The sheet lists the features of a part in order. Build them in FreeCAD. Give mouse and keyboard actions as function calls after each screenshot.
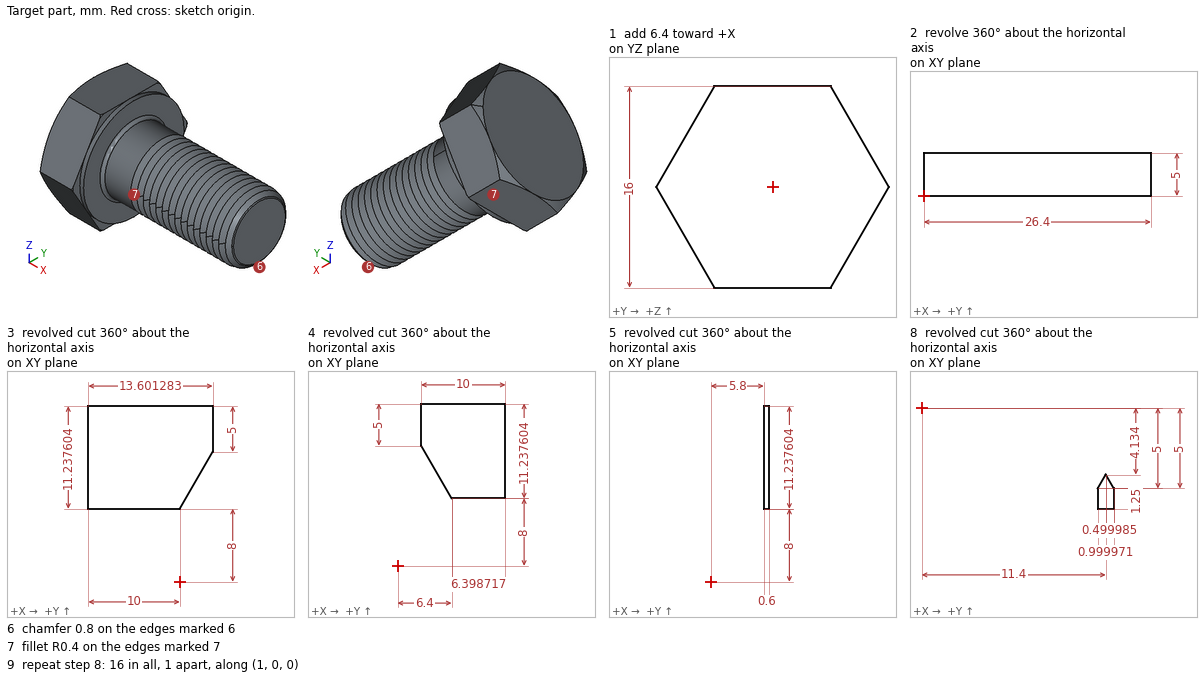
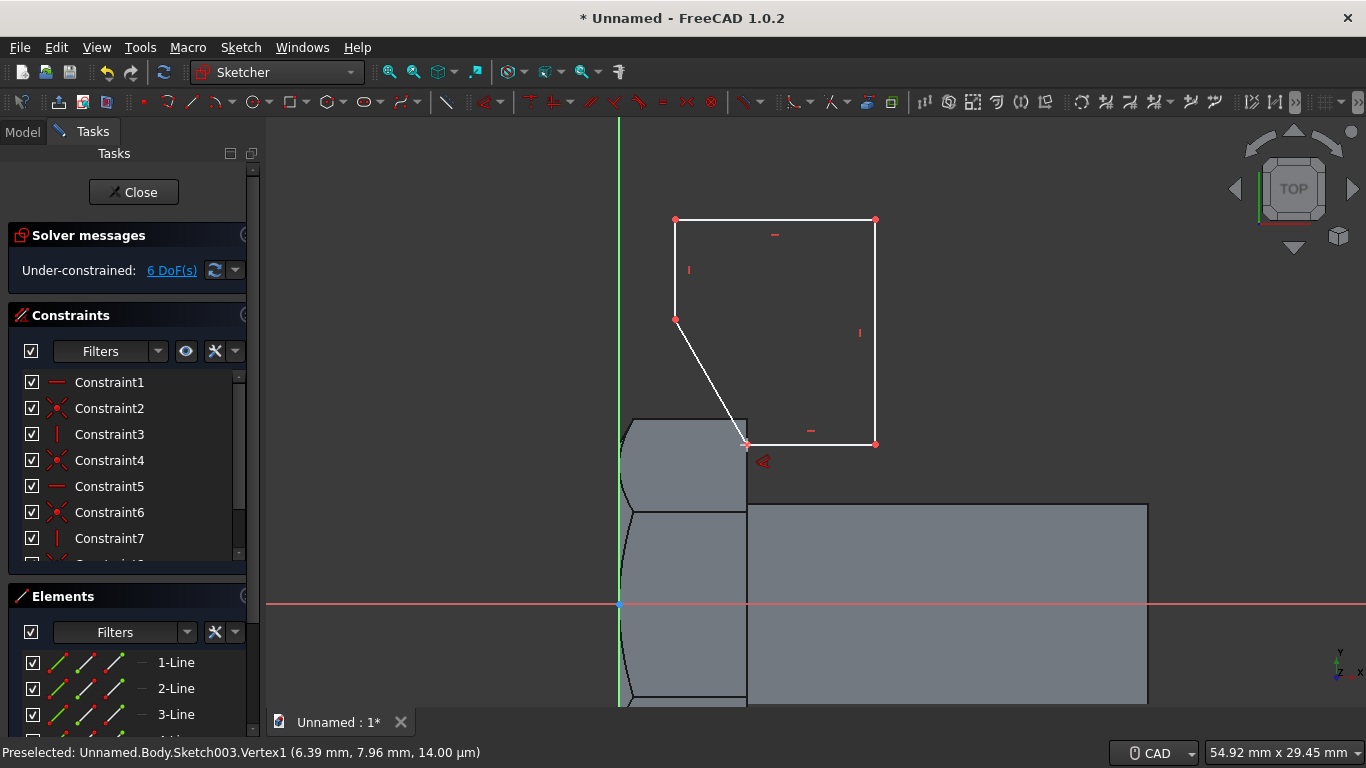
click(675, 250)
click(641, 270)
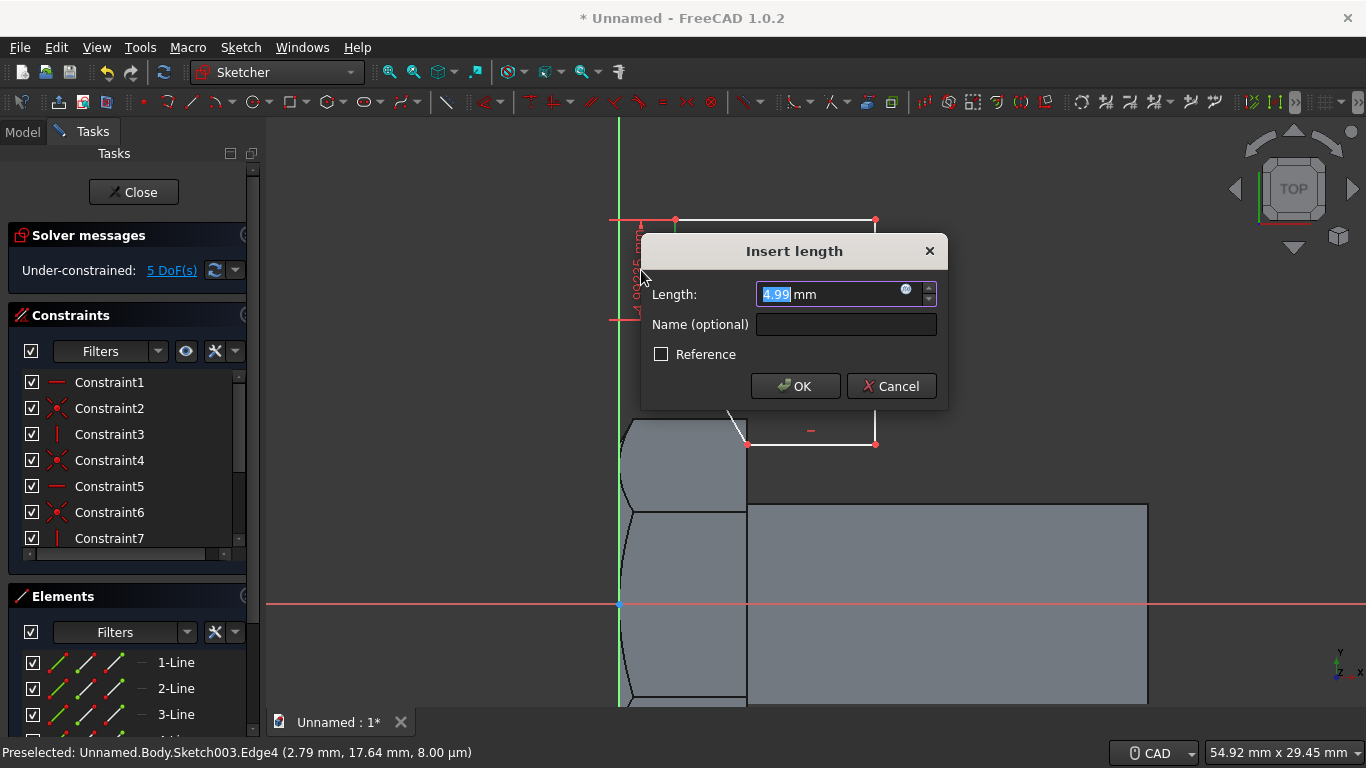
text(5)
key(Return)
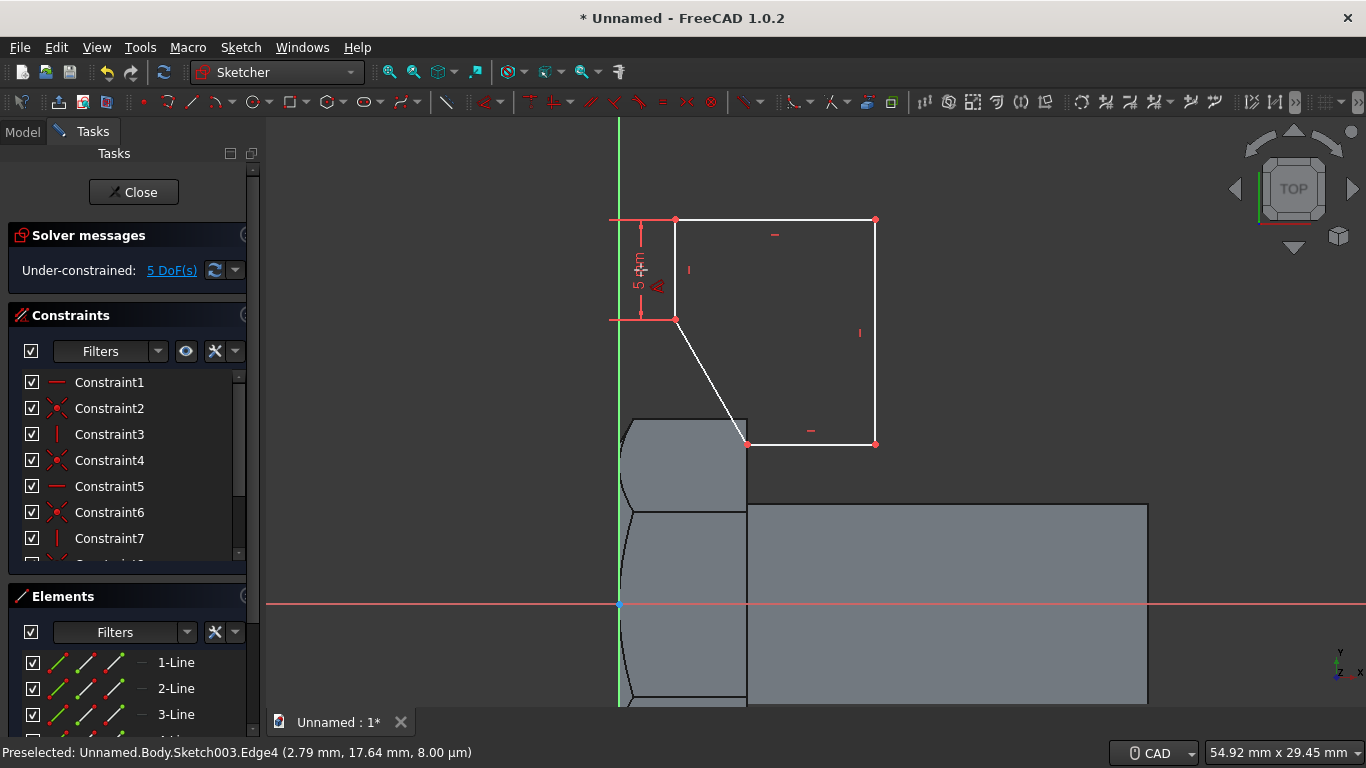
click(815, 220)
click(775, 186)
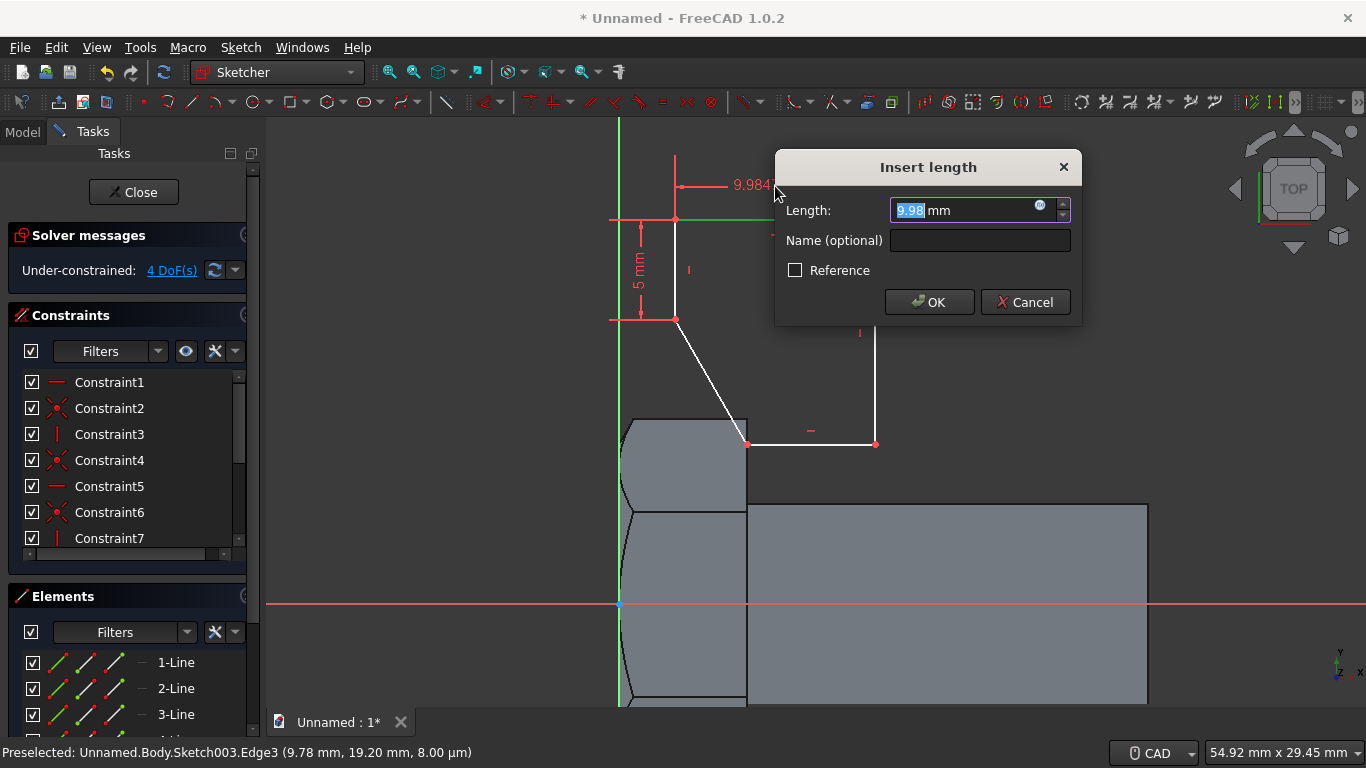
text(10)
key(Return)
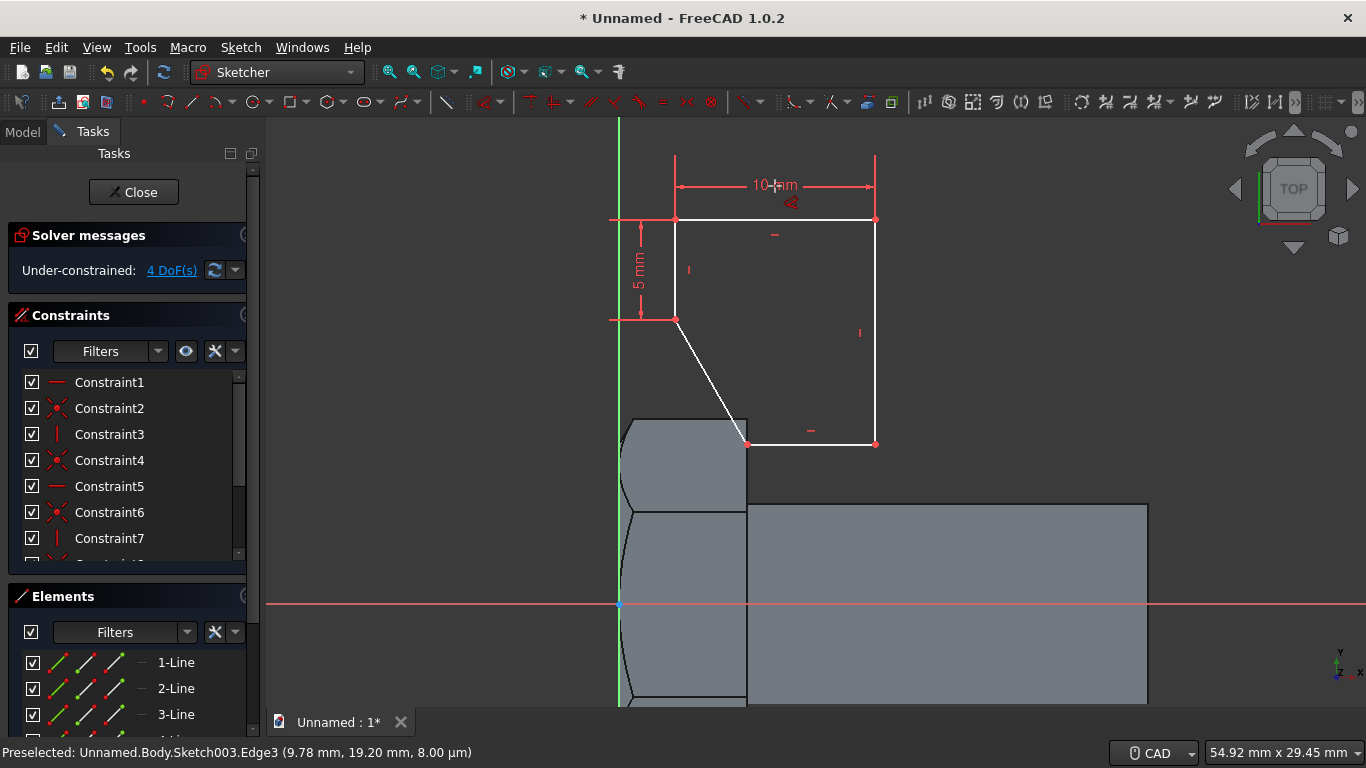
click(747, 445)
click(585, 525)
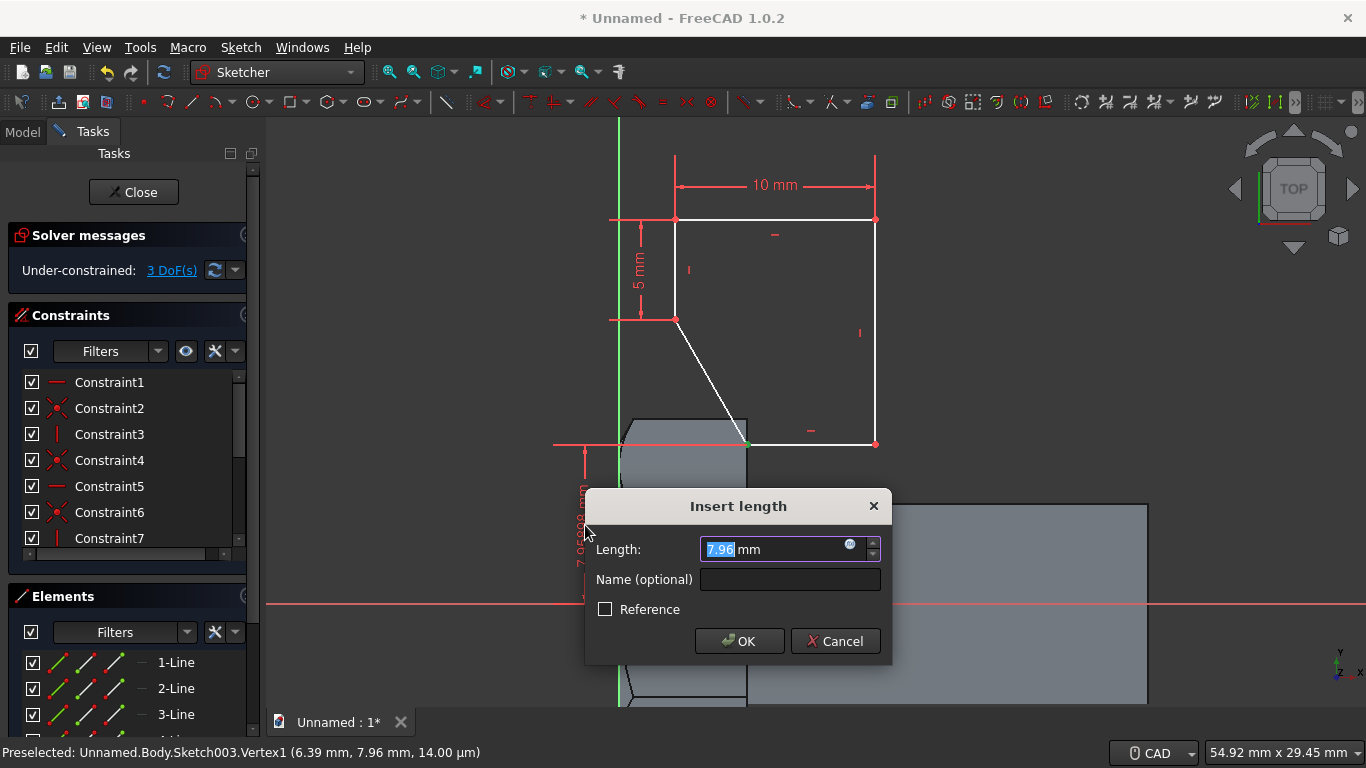
text(8)
key(Return)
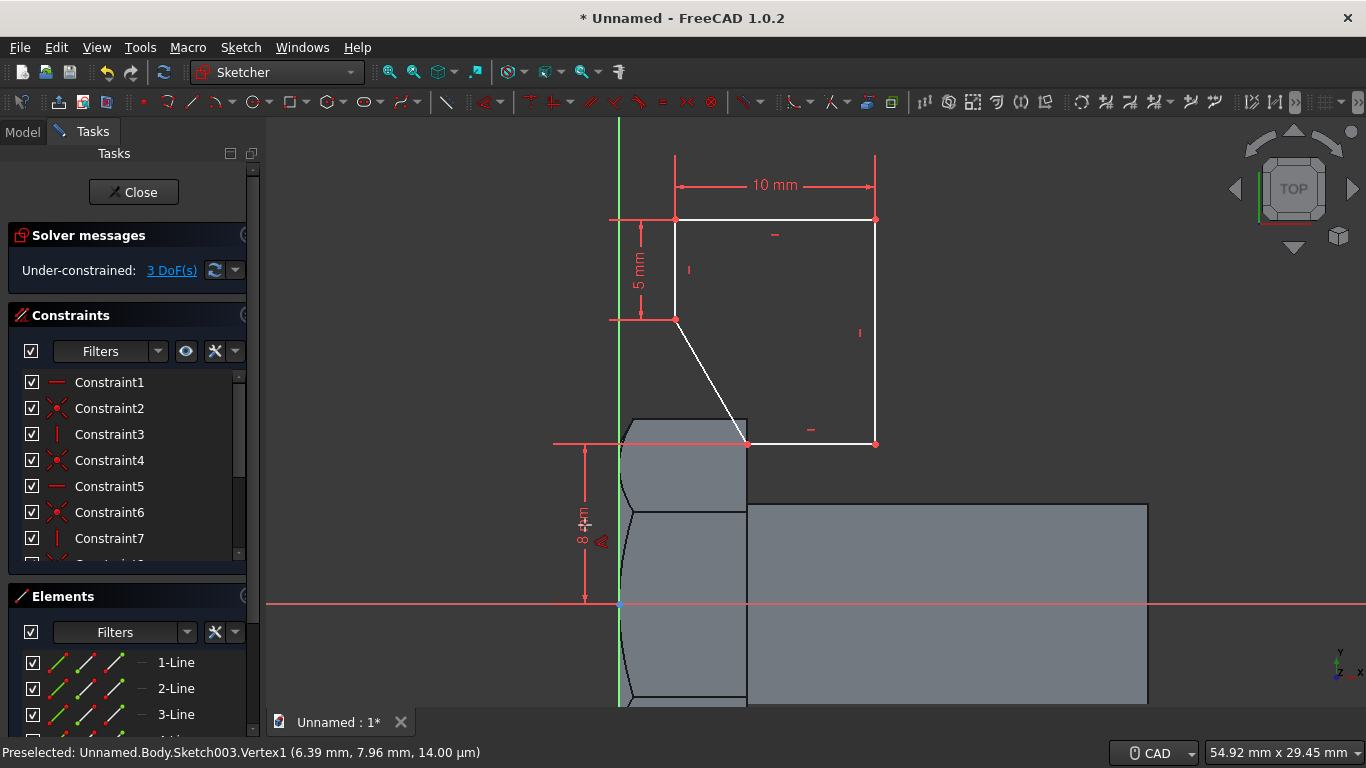
click(747, 444)
click(683, 638)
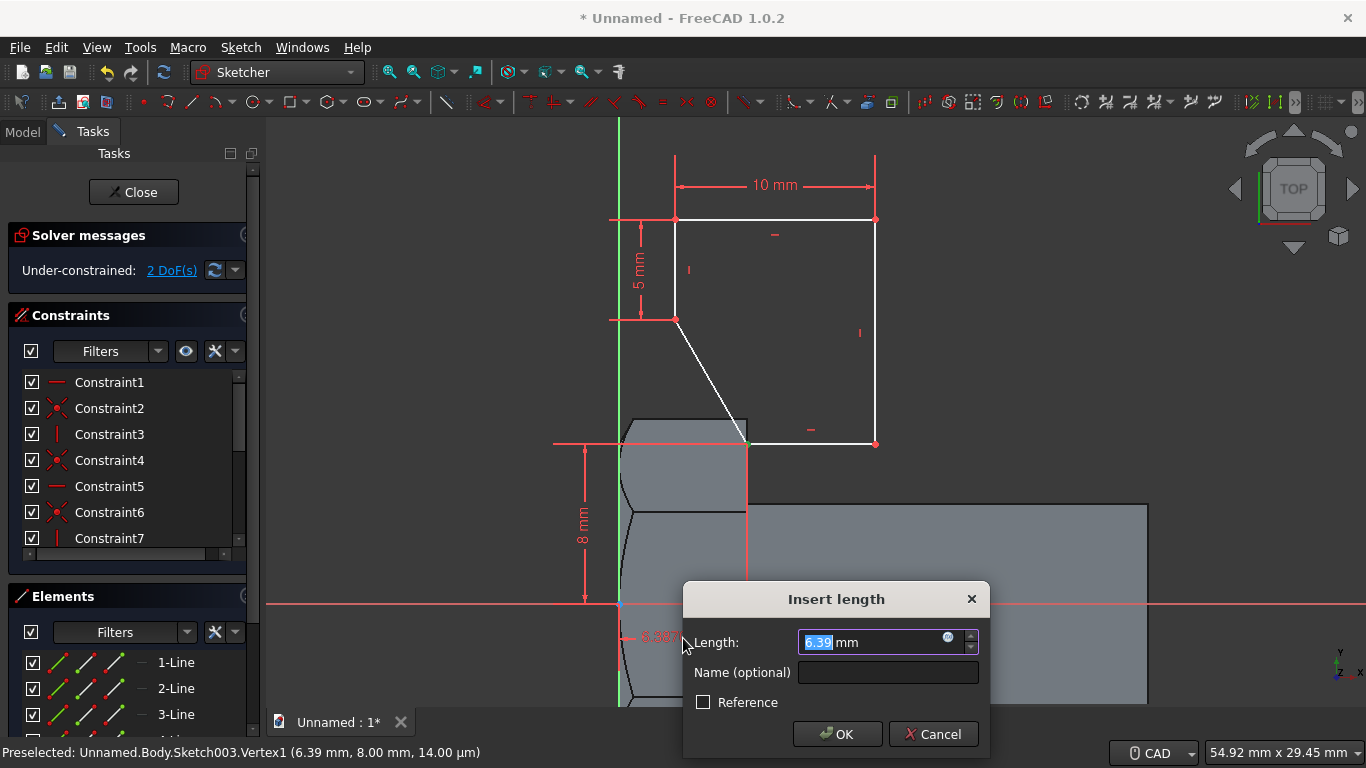
text(6.4)
key(Return)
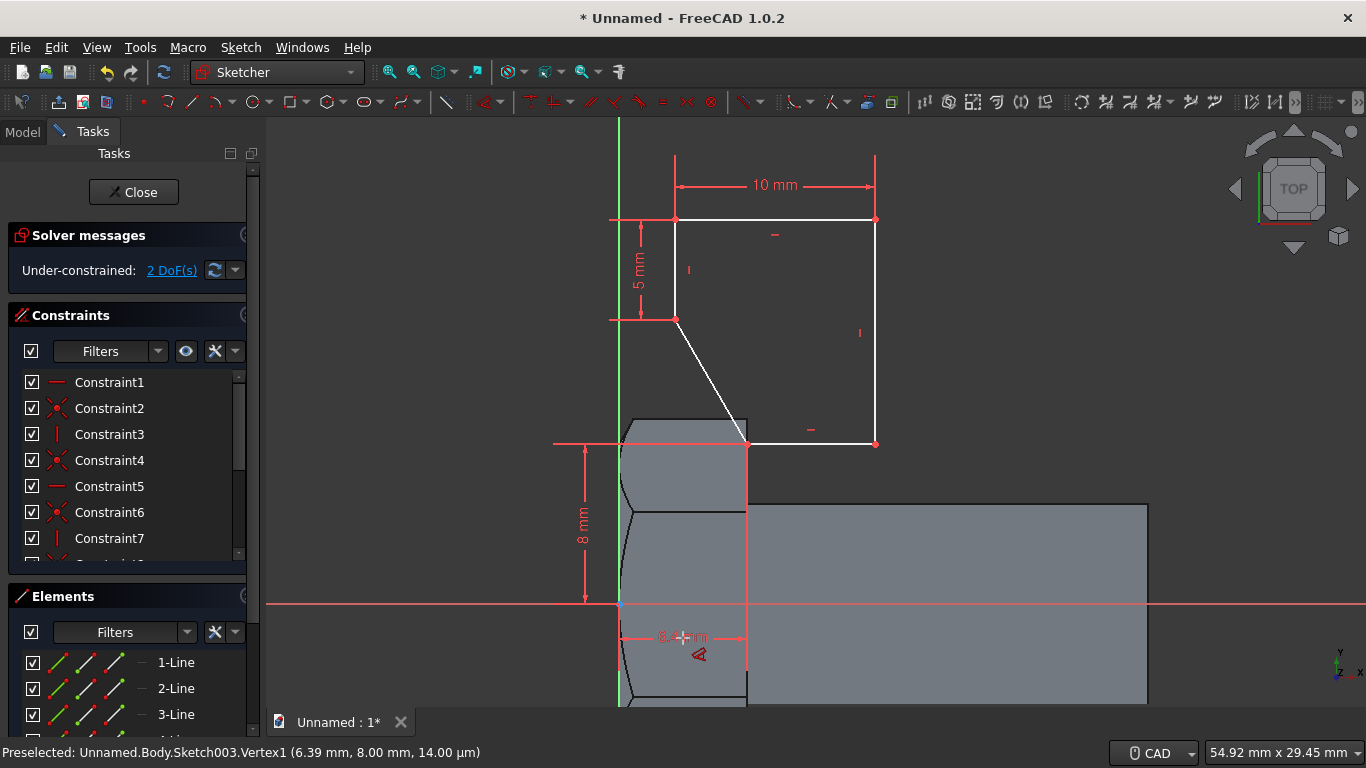
click(786, 444)
click(811, 478)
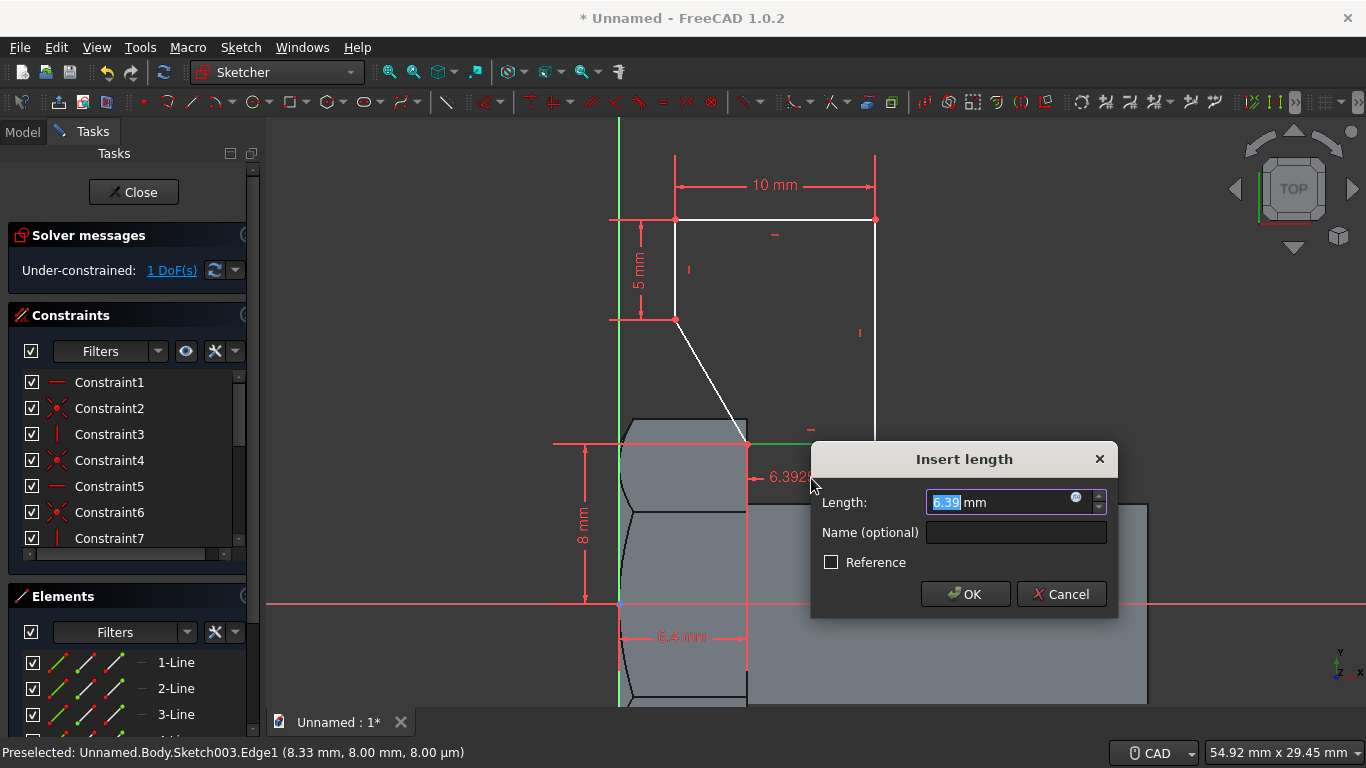
text(6.398717)
key(Return)